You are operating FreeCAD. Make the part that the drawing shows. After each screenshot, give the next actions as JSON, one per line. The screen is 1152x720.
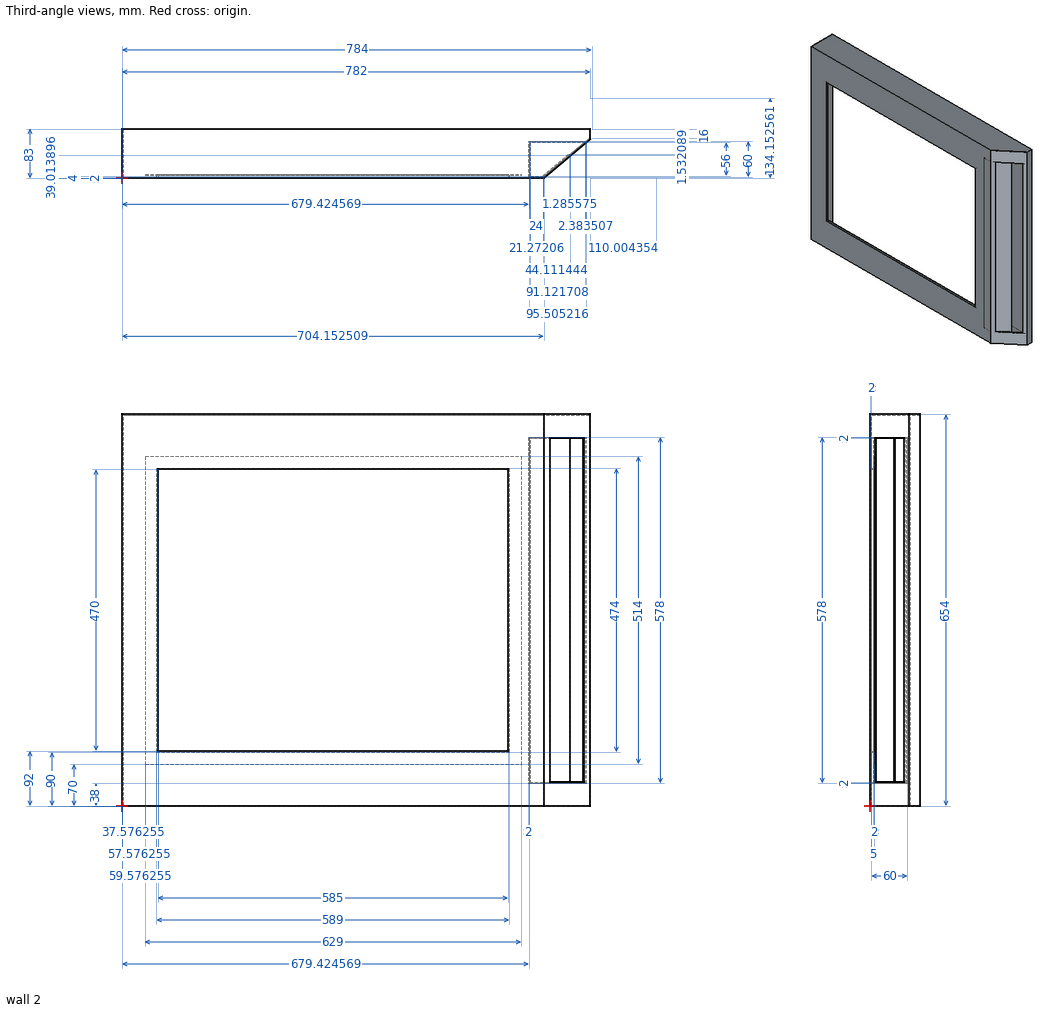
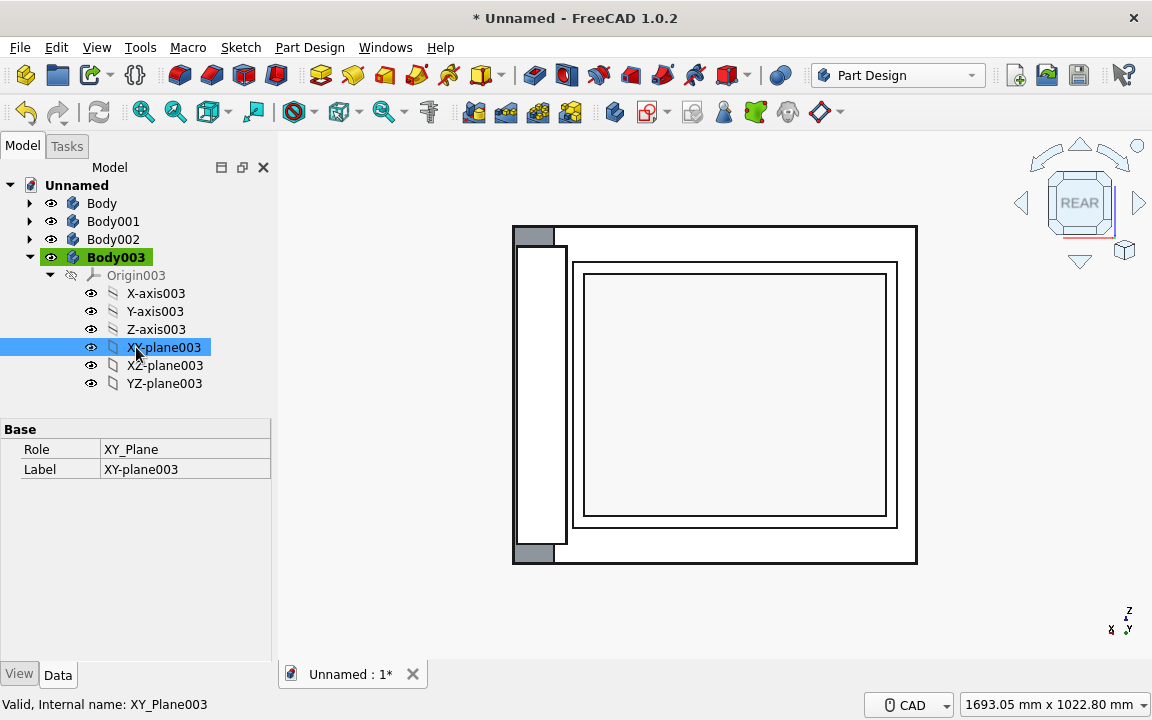
{"action": "left_click", "coordinate": [820, 112]}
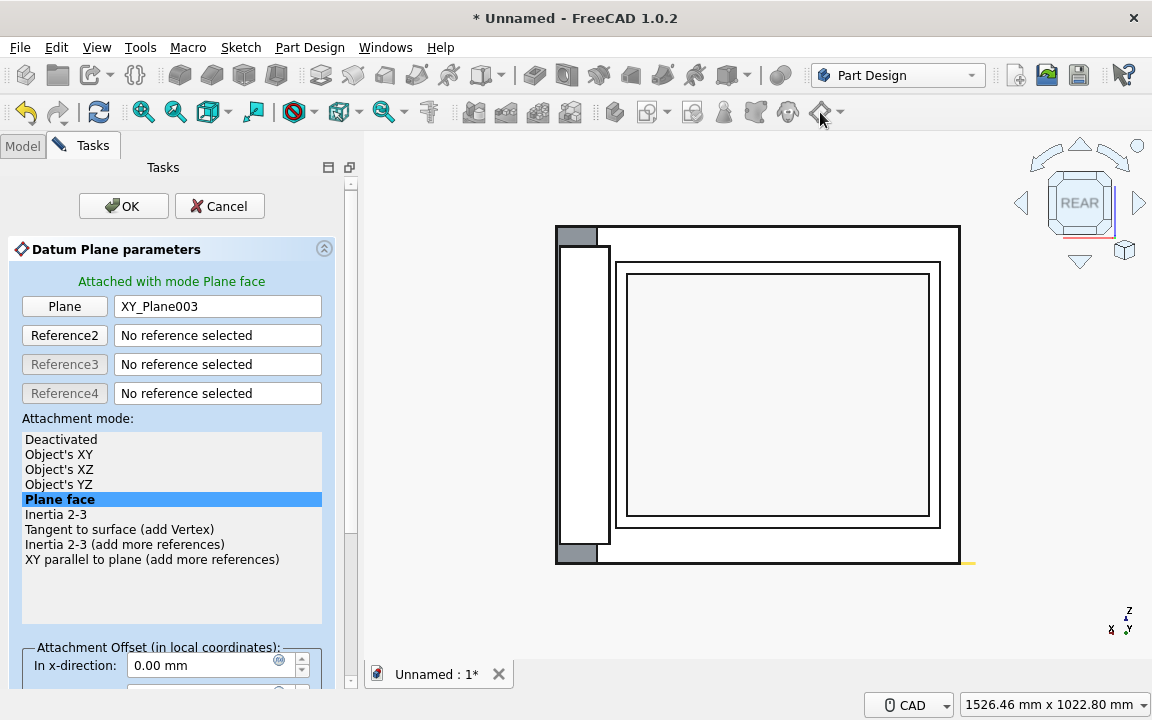
{"action": "scroll", "coordinate": [351, 432], "scroll_direction": "down", "scroll_amount": 2}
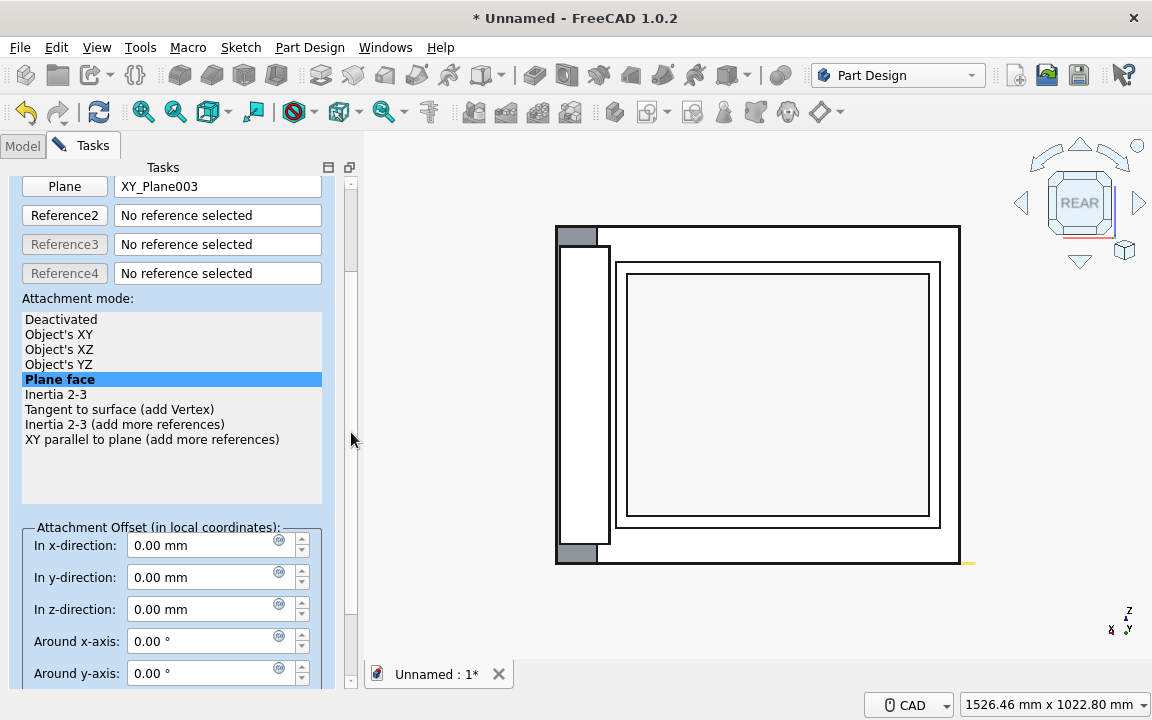
{"action": "triple_click", "coordinate": [210, 609]}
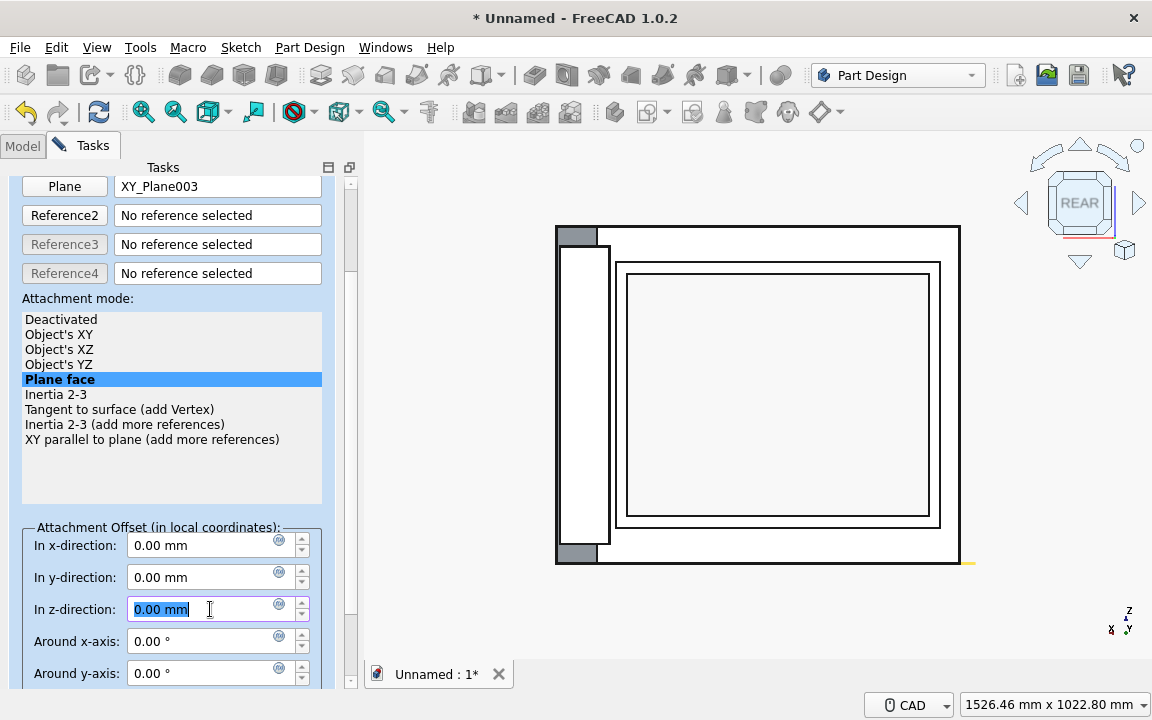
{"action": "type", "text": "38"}
{"action": "key", "text": "Tab"}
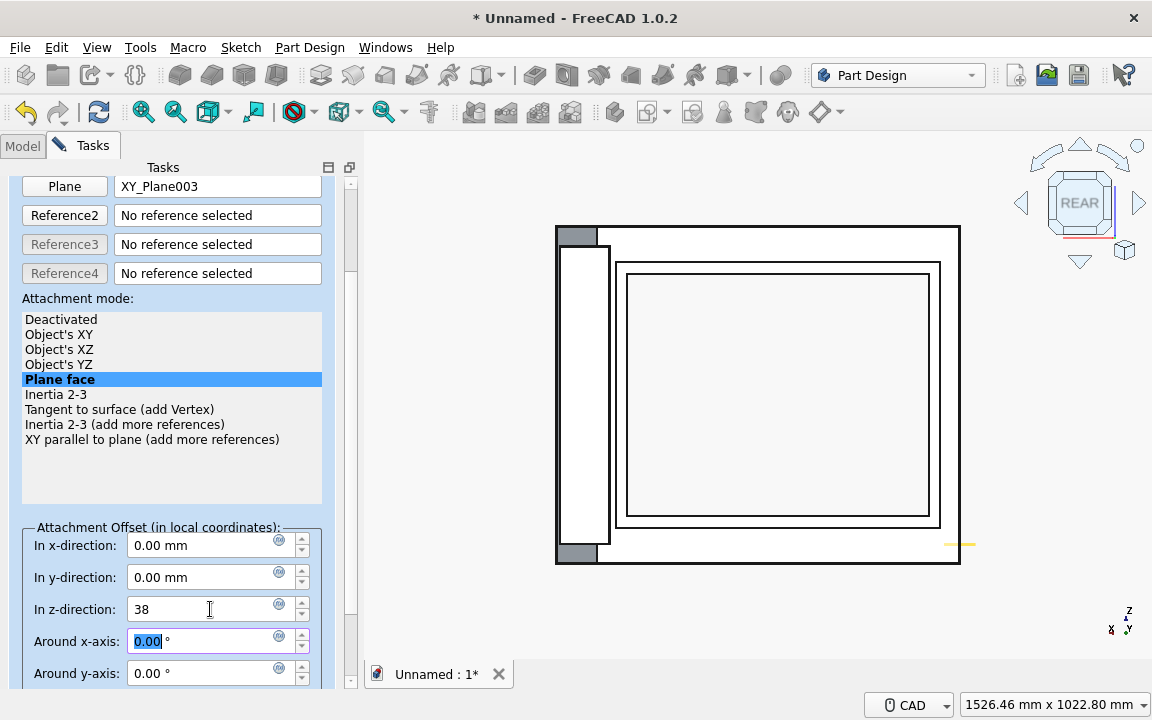
{"action": "scroll", "coordinate": [351, 432], "scroll_direction": "up", "scroll_amount": 3}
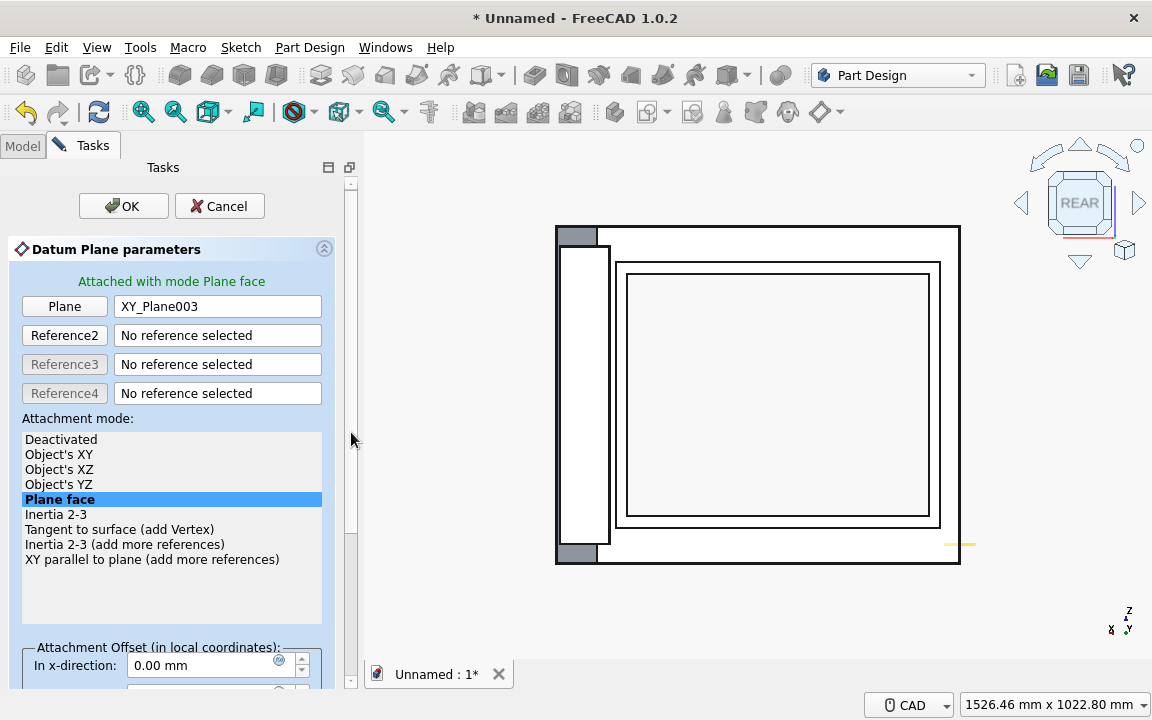
{"action": "left_click", "coordinate": [124, 206]}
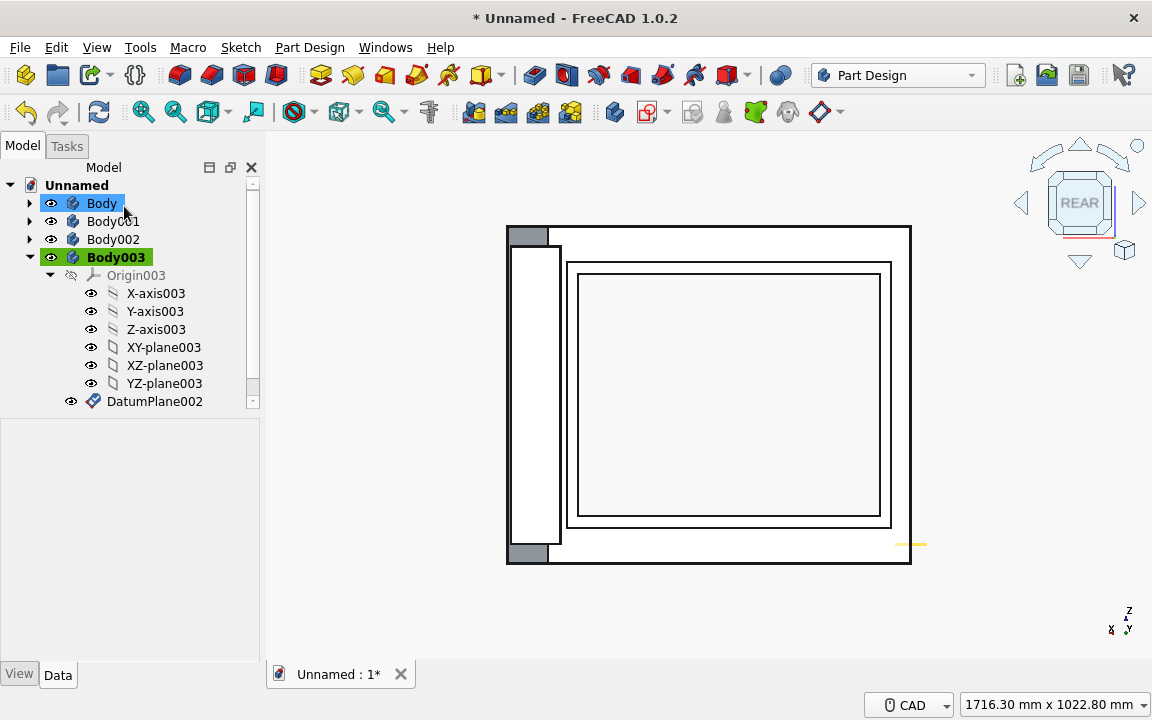
{"action": "left_click", "coordinate": [116, 401]}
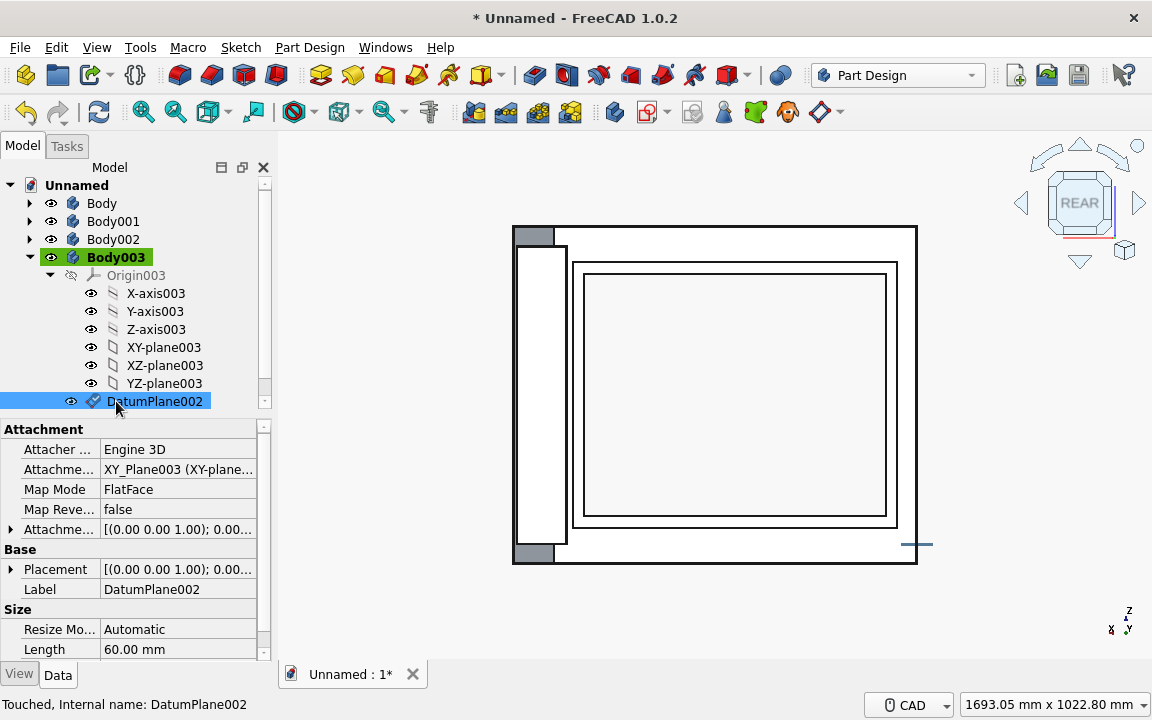
{"action": "left_click", "coordinate": [648, 112]}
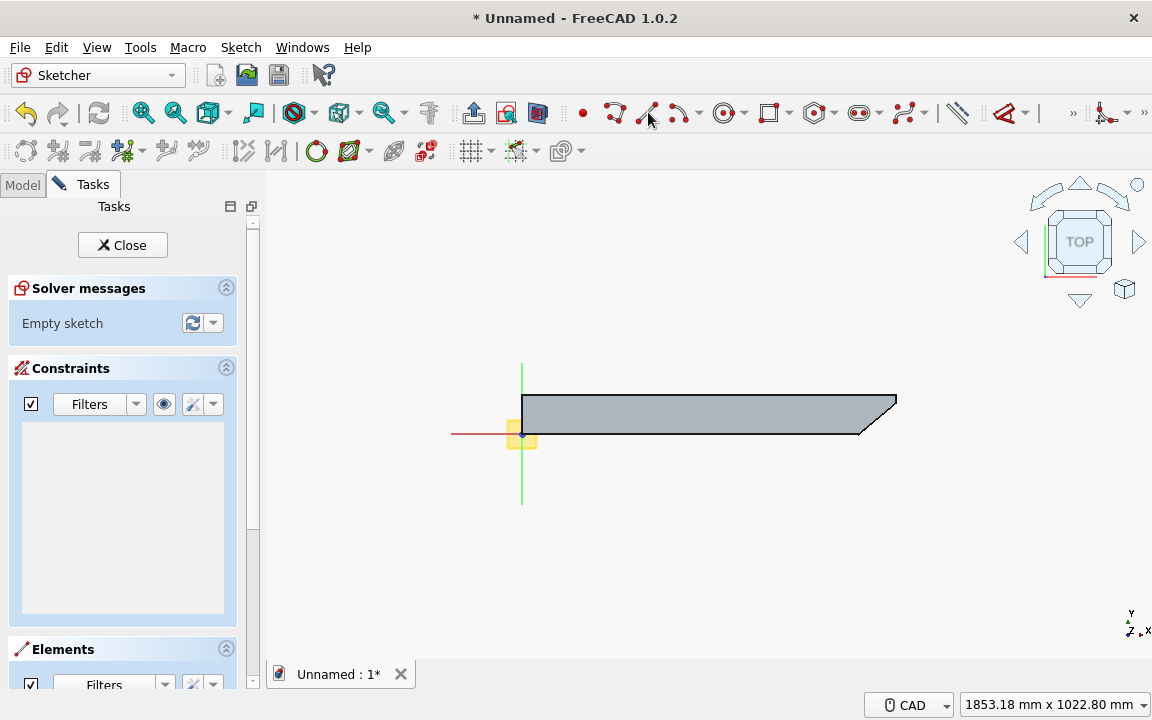
{"action": "scroll", "coordinate": [893, 419], "scroll_direction": "up", "scroll_amount": 12}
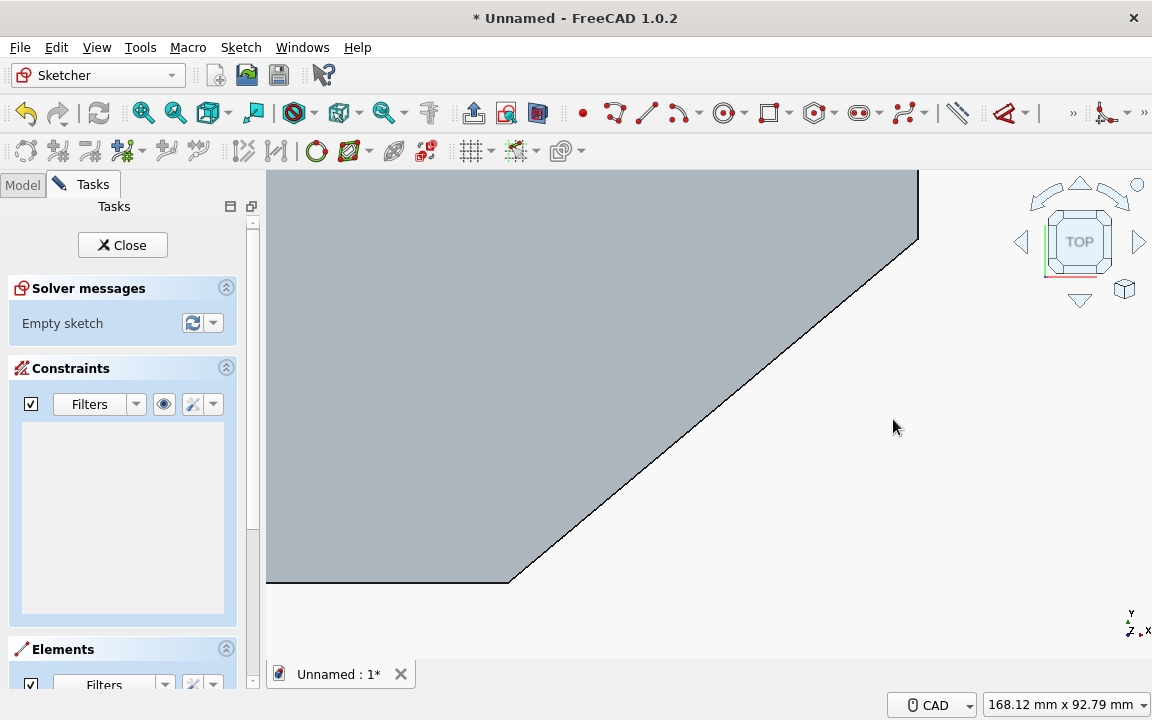
{"action": "left_click", "coordinate": [616, 114]}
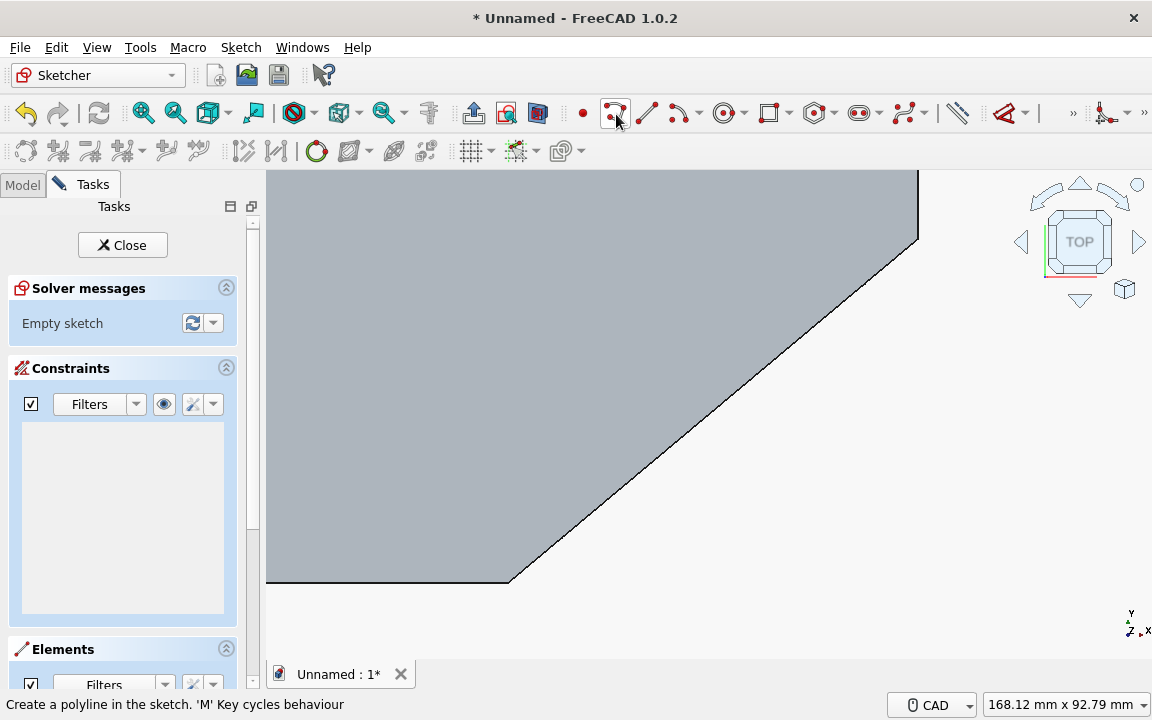
{"action": "scroll", "coordinate": [378, 572], "scroll_direction": "up", "scroll_amount": 3}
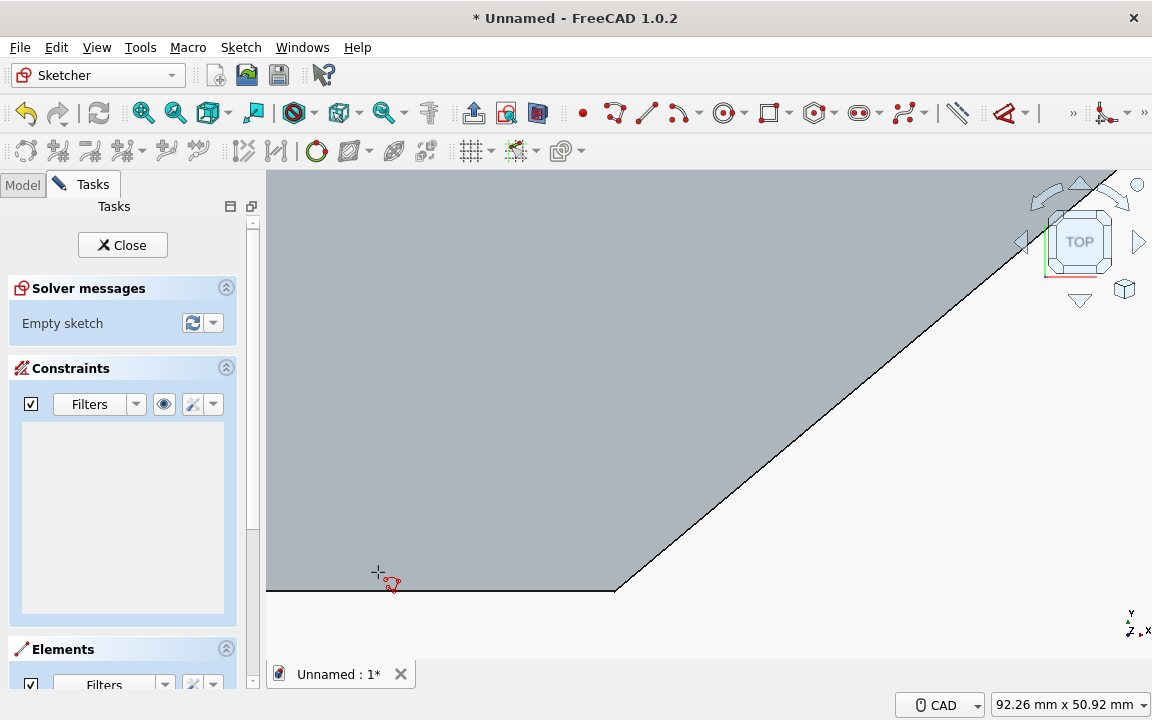
{"action": "left_click", "coordinate": [377, 572]}